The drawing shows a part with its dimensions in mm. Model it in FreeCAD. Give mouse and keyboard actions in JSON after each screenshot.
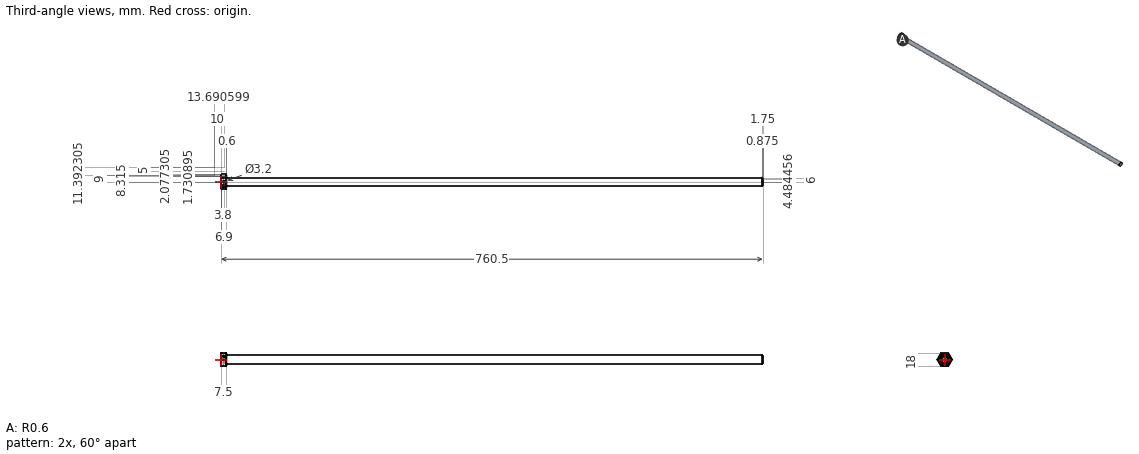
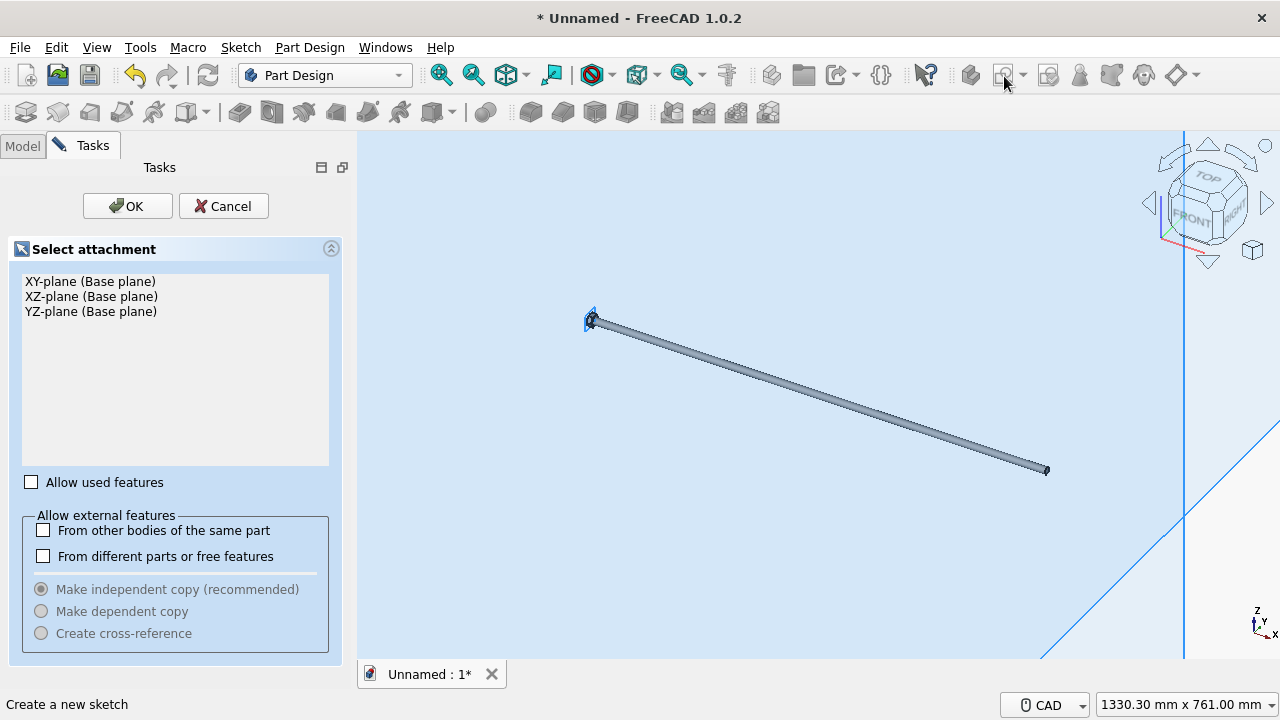
{"action": "left_click", "coordinate": [82, 282]}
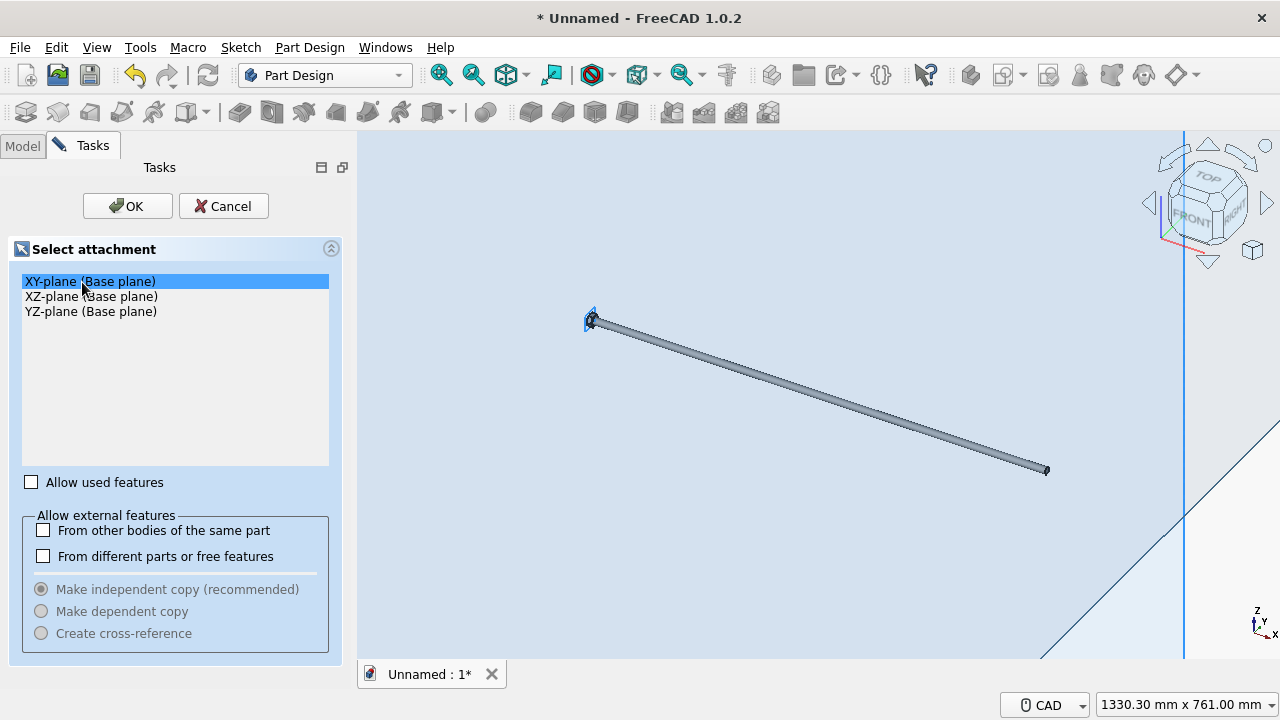
{"action": "left_click", "coordinate": [128, 206]}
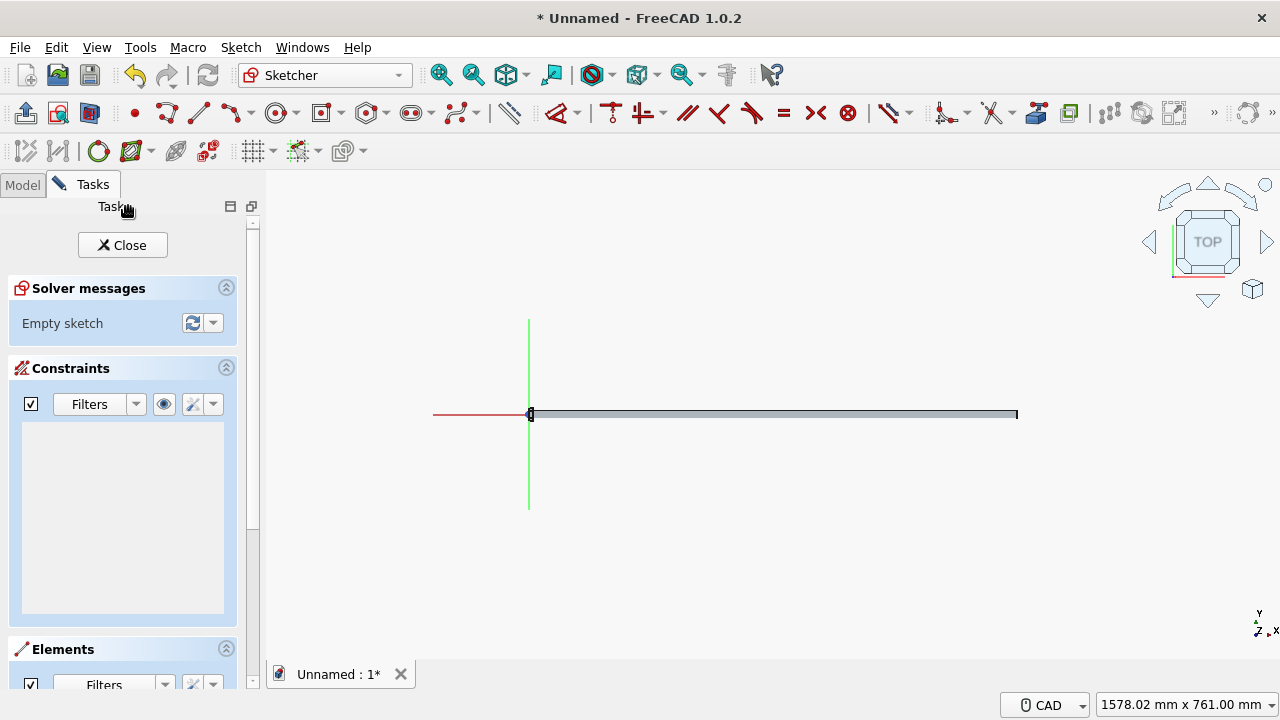
{"action": "key", "text": "q s"}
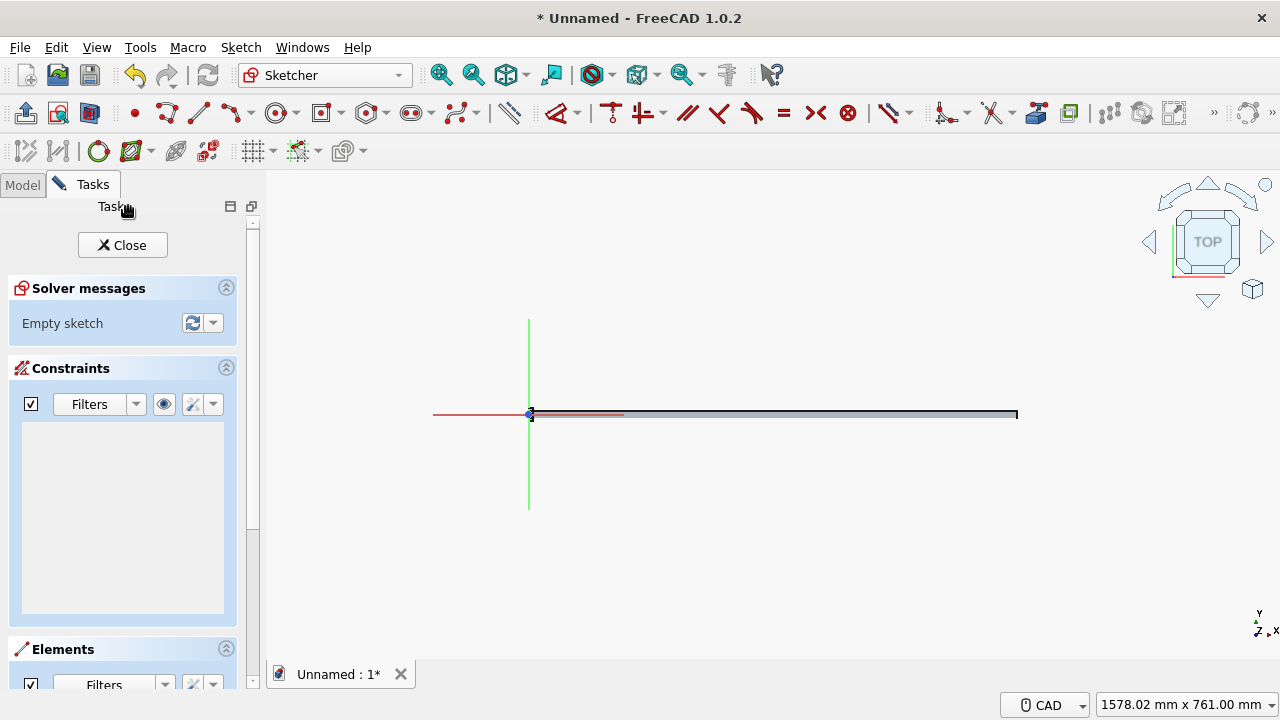
{"action": "scroll", "coordinate": [524, 408], "scroll_direction": "up", "scroll_amount": 15}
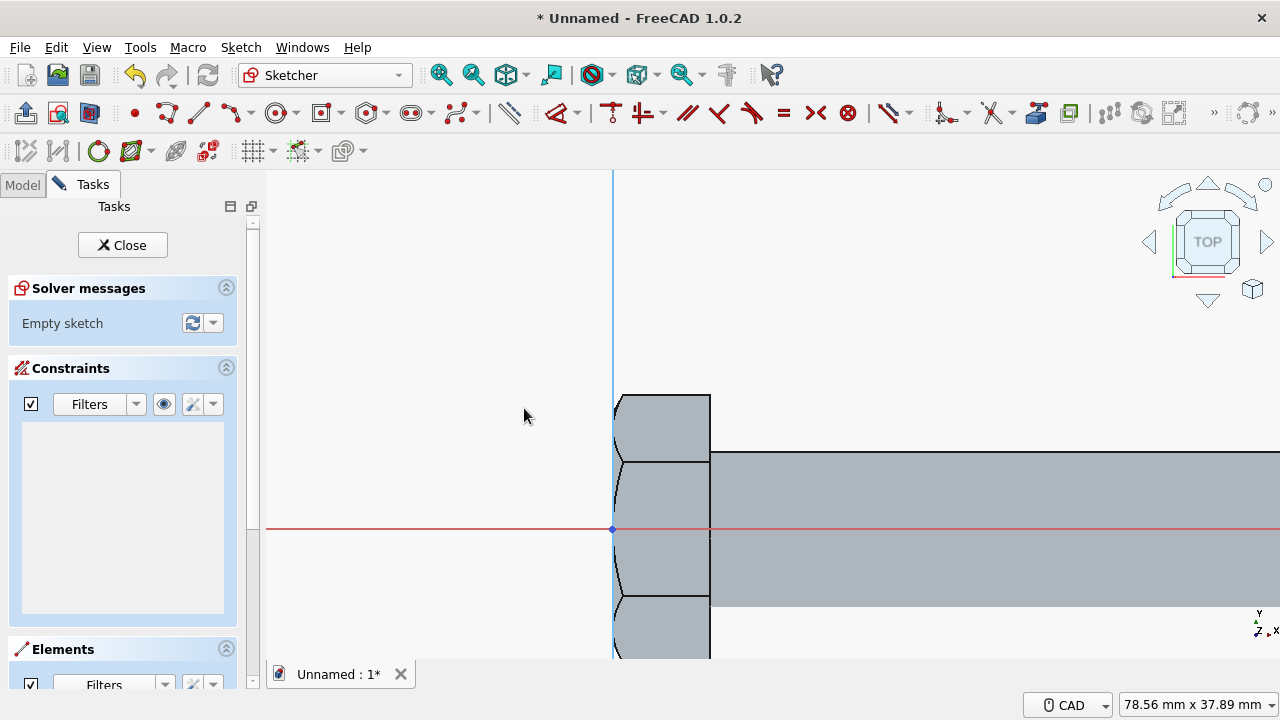
{"action": "scroll", "coordinate": [706, 408], "scroll_direction": "up", "scroll_amount": 12}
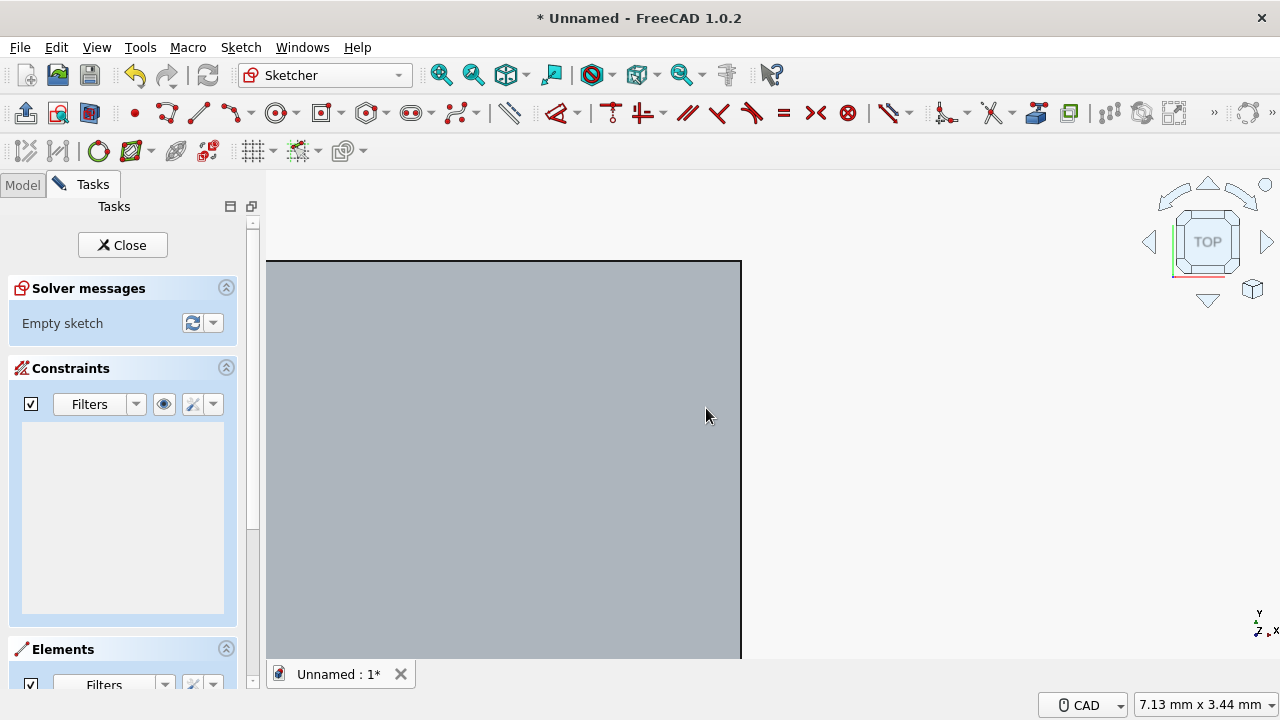
{"action": "key", "text": "g m"}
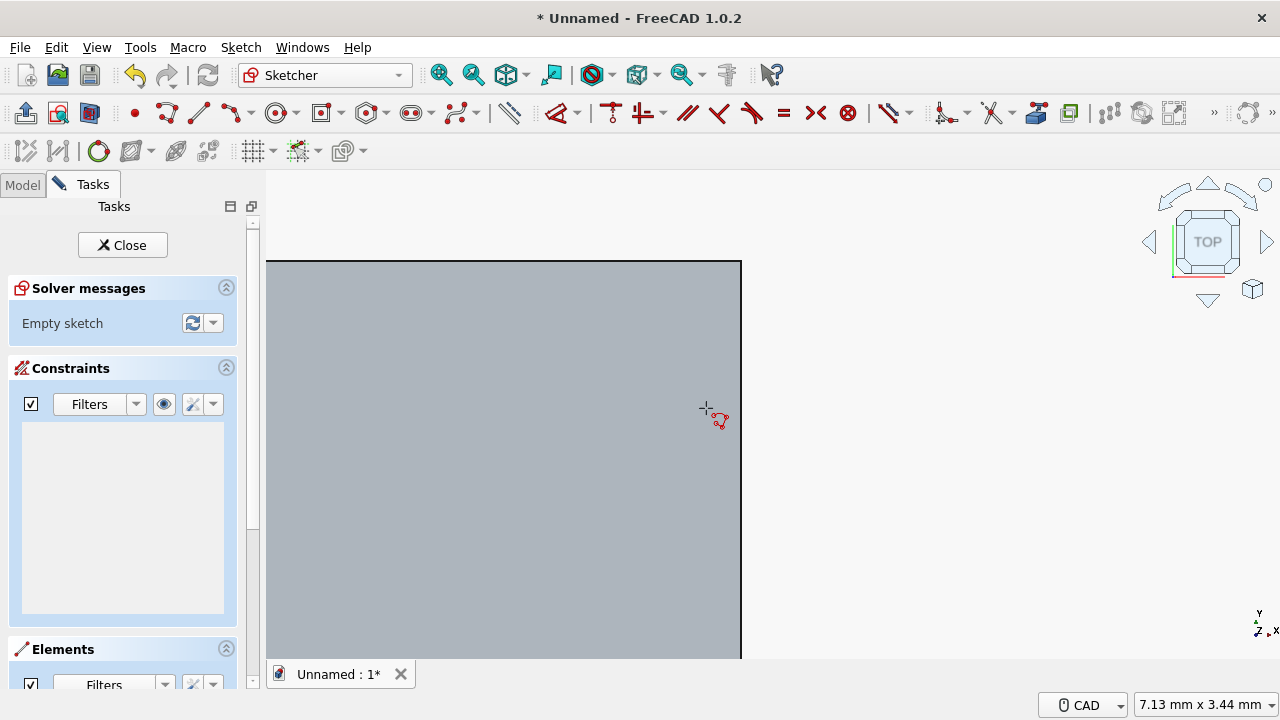
{"action": "left_click", "coordinate": [655, 507]}
{"action": "left_click", "coordinate": [741, 557]}
{"action": "left_click", "coordinate": [741, 261]}
{"action": "left_click", "coordinate": [655, 261]}
{"action": "left_click", "coordinate": [655, 508]}
{"action": "key", "text": "Escape"}
{"action": "key", "text": "Escape"}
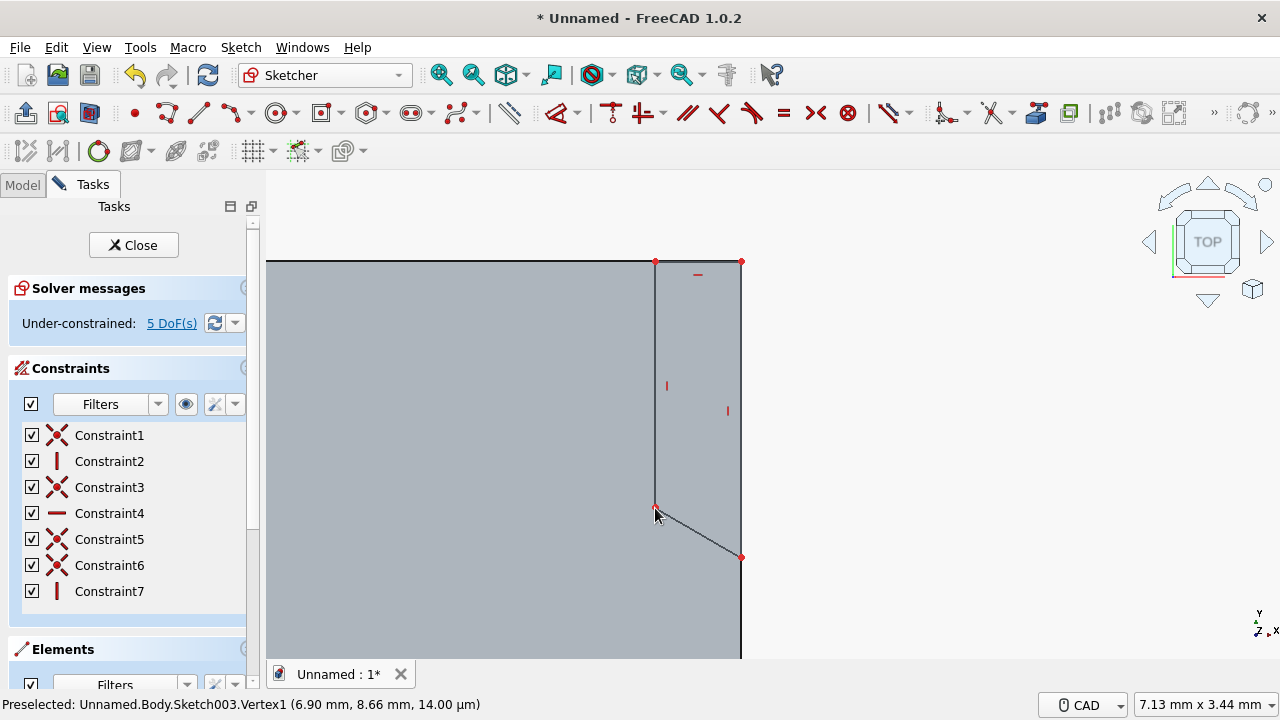
{"action": "key", "text": "d"}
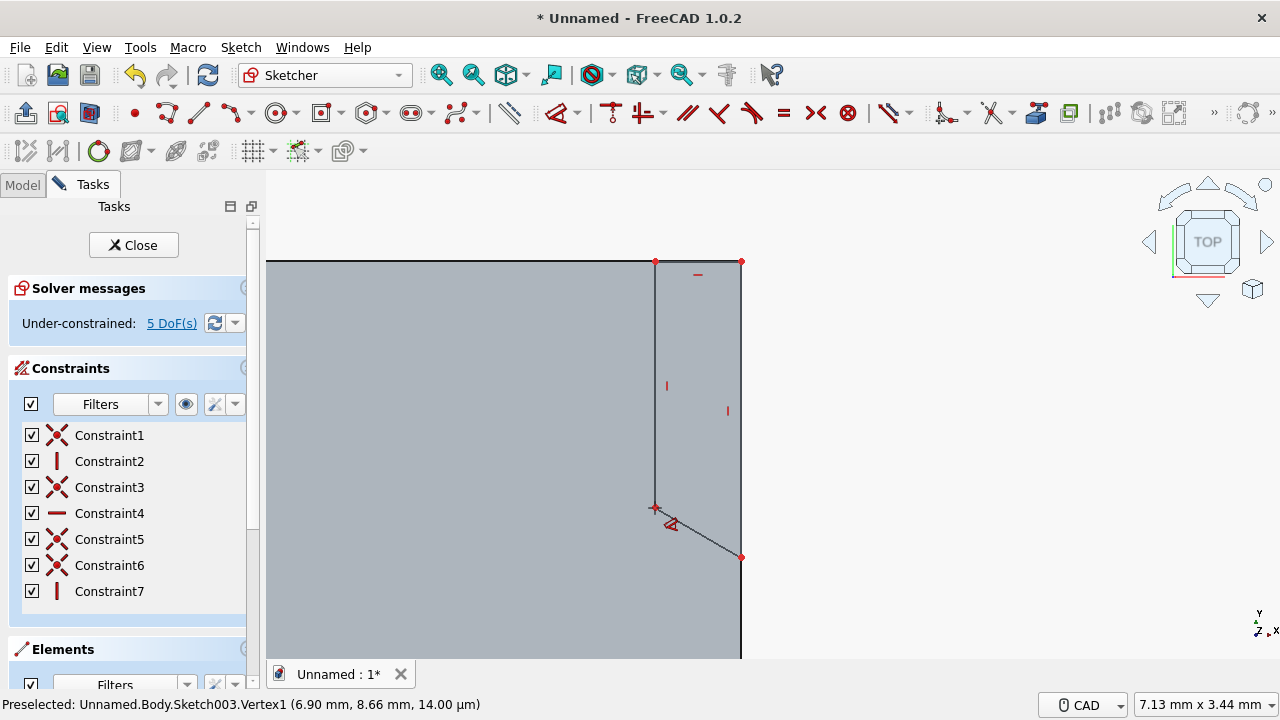
{"action": "left_click", "coordinate": [715, 262]}
{"action": "left_click", "coordinate": [698, 228]}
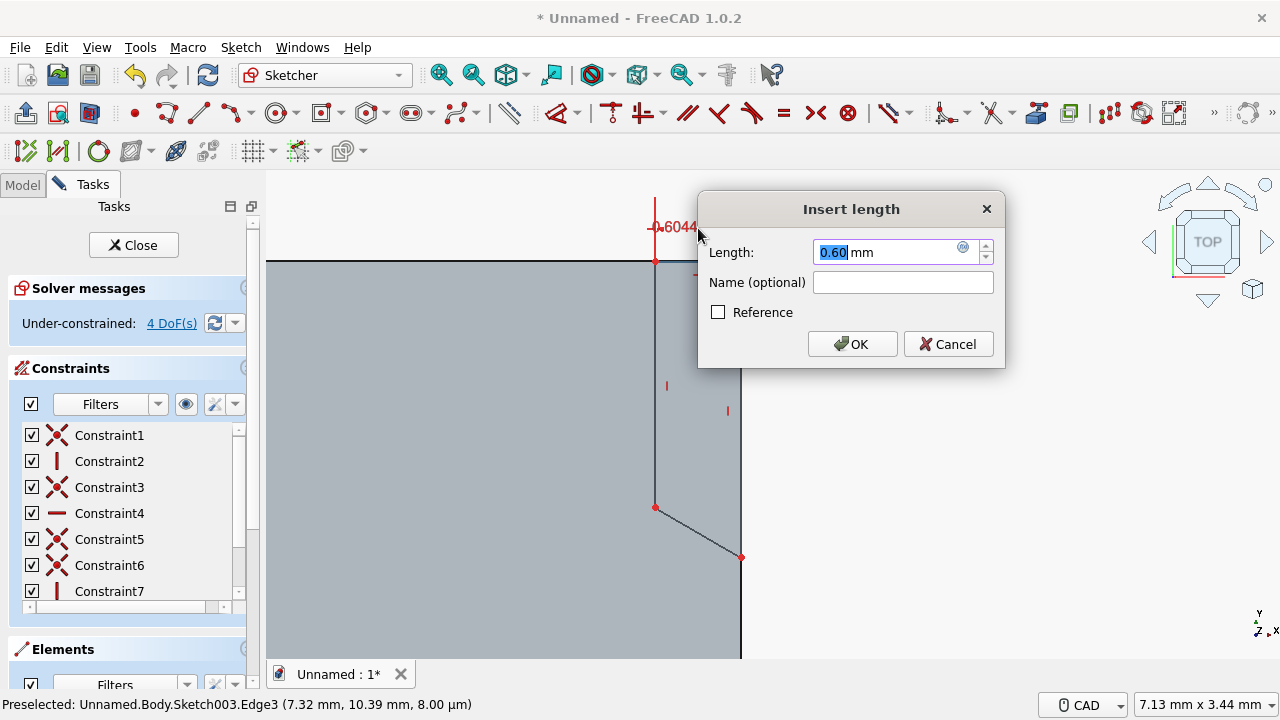
{"action": "type", "text": "0.6"}
{"action": "key", "text": "Return"}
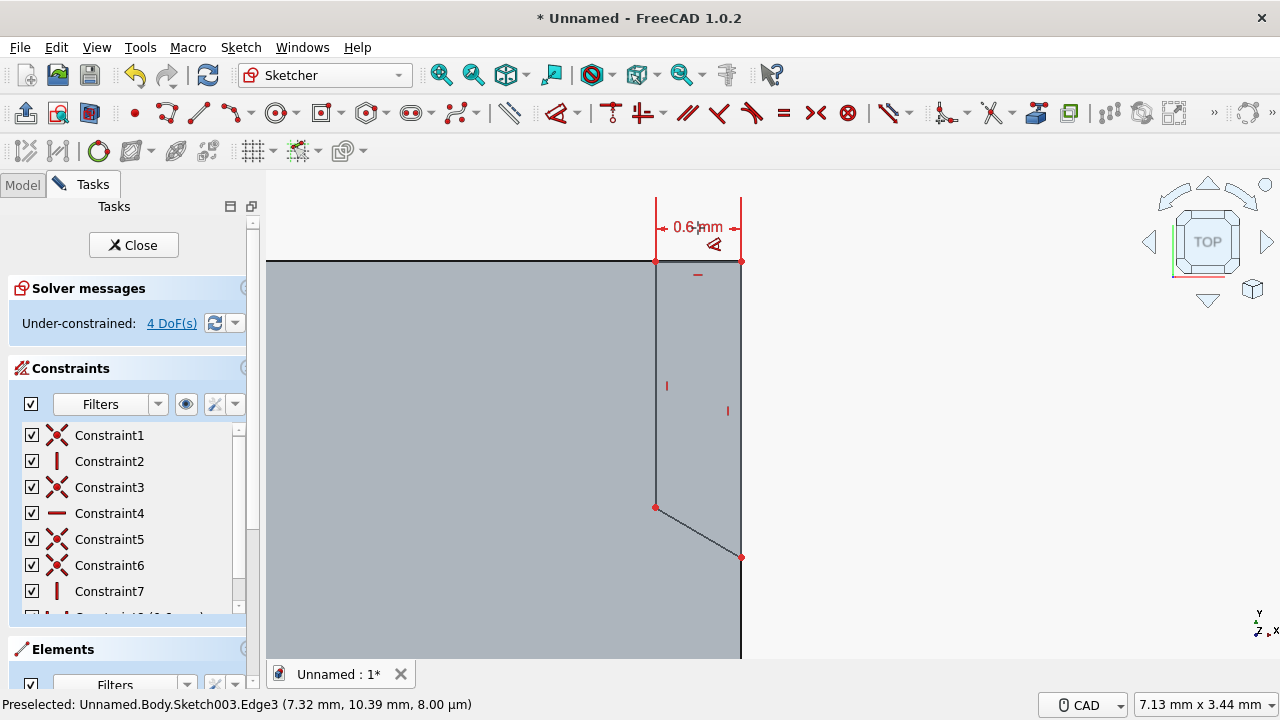
{"action": "left_click", "coordinate": [656, 508]}
{"action": "left_click", "coordinate": [475, 474]}